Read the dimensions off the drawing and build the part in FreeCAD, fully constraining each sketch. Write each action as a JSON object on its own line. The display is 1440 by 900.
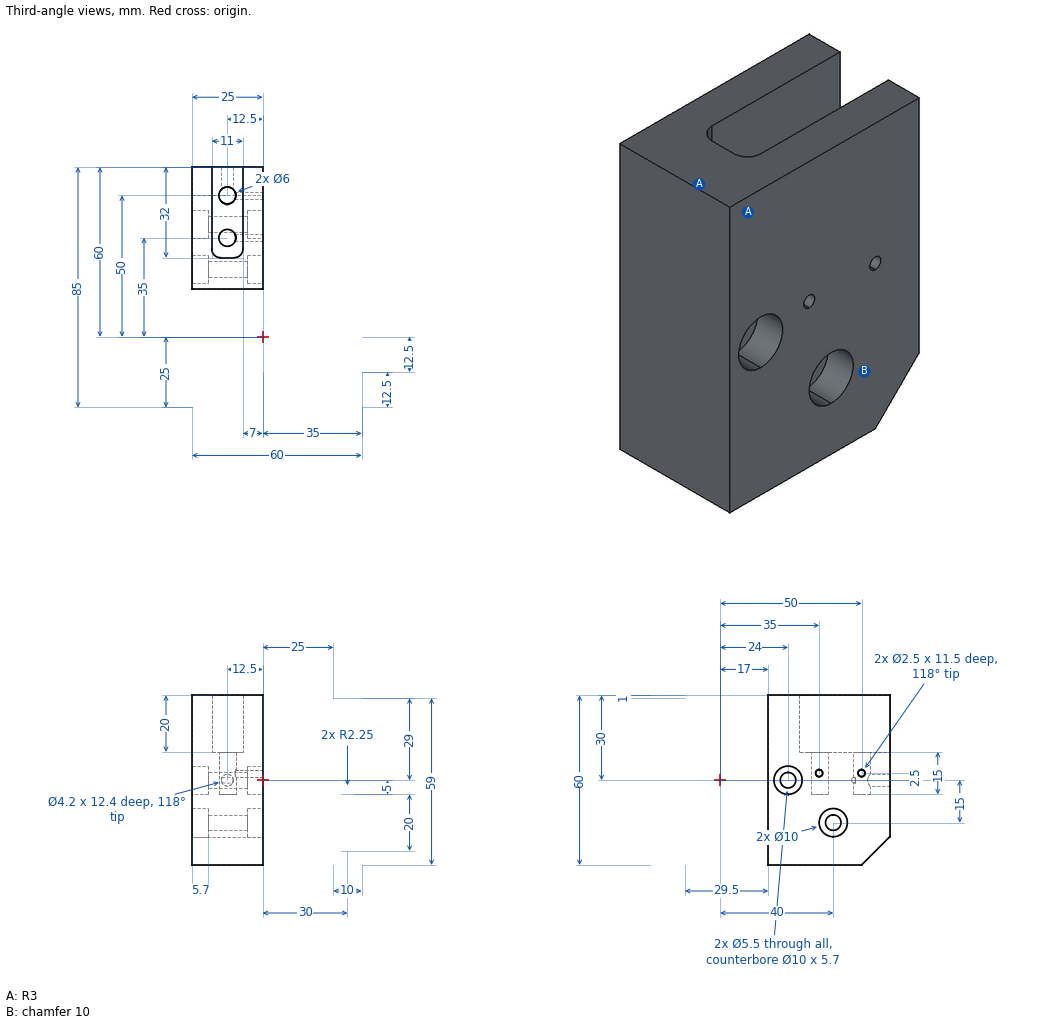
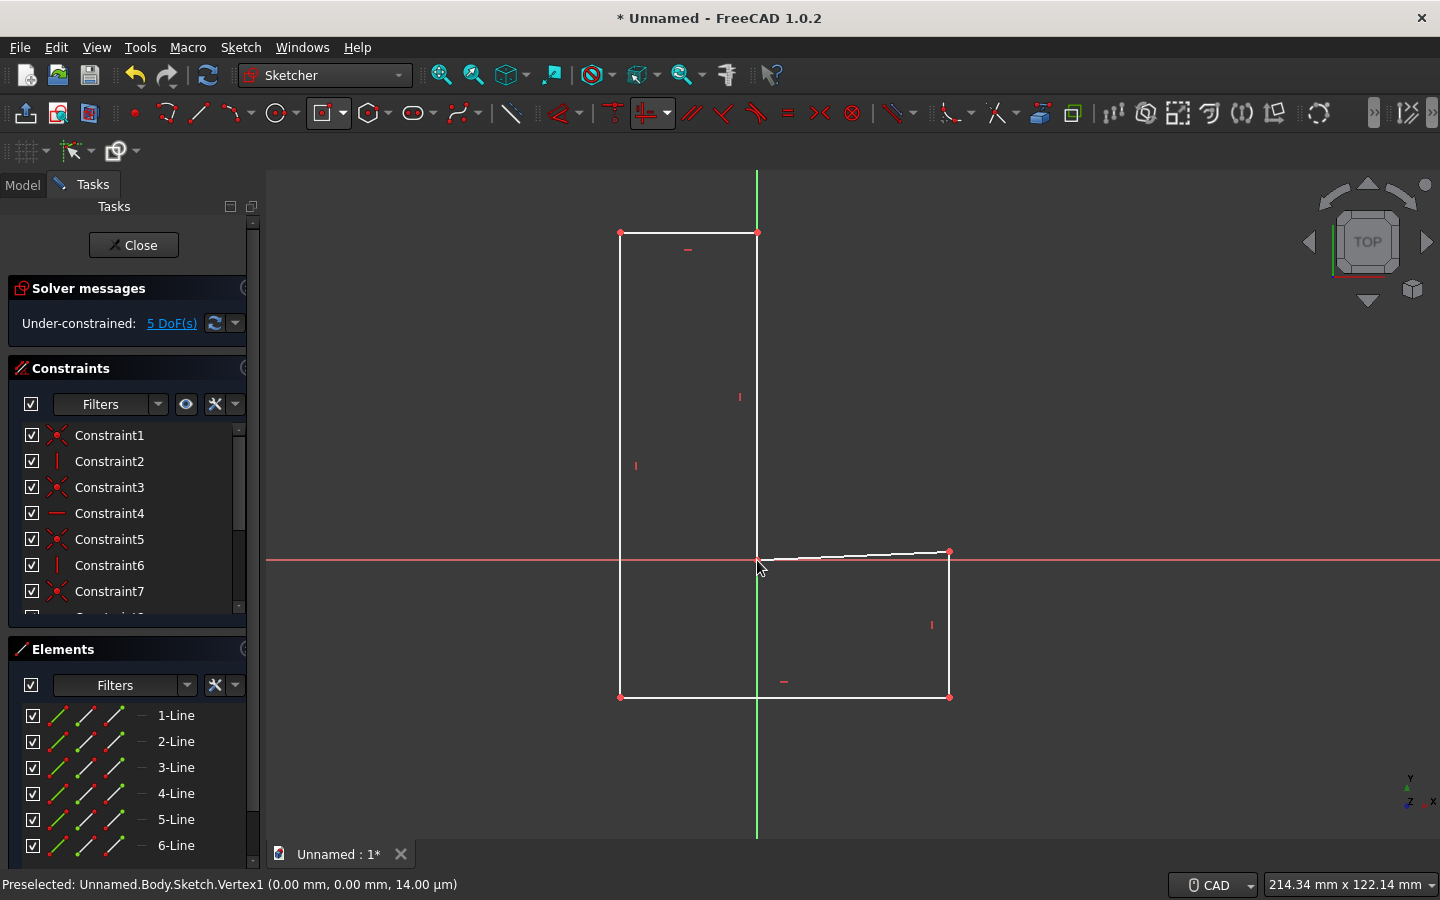
{"action": "left_click", "coordinate": [815, 558]}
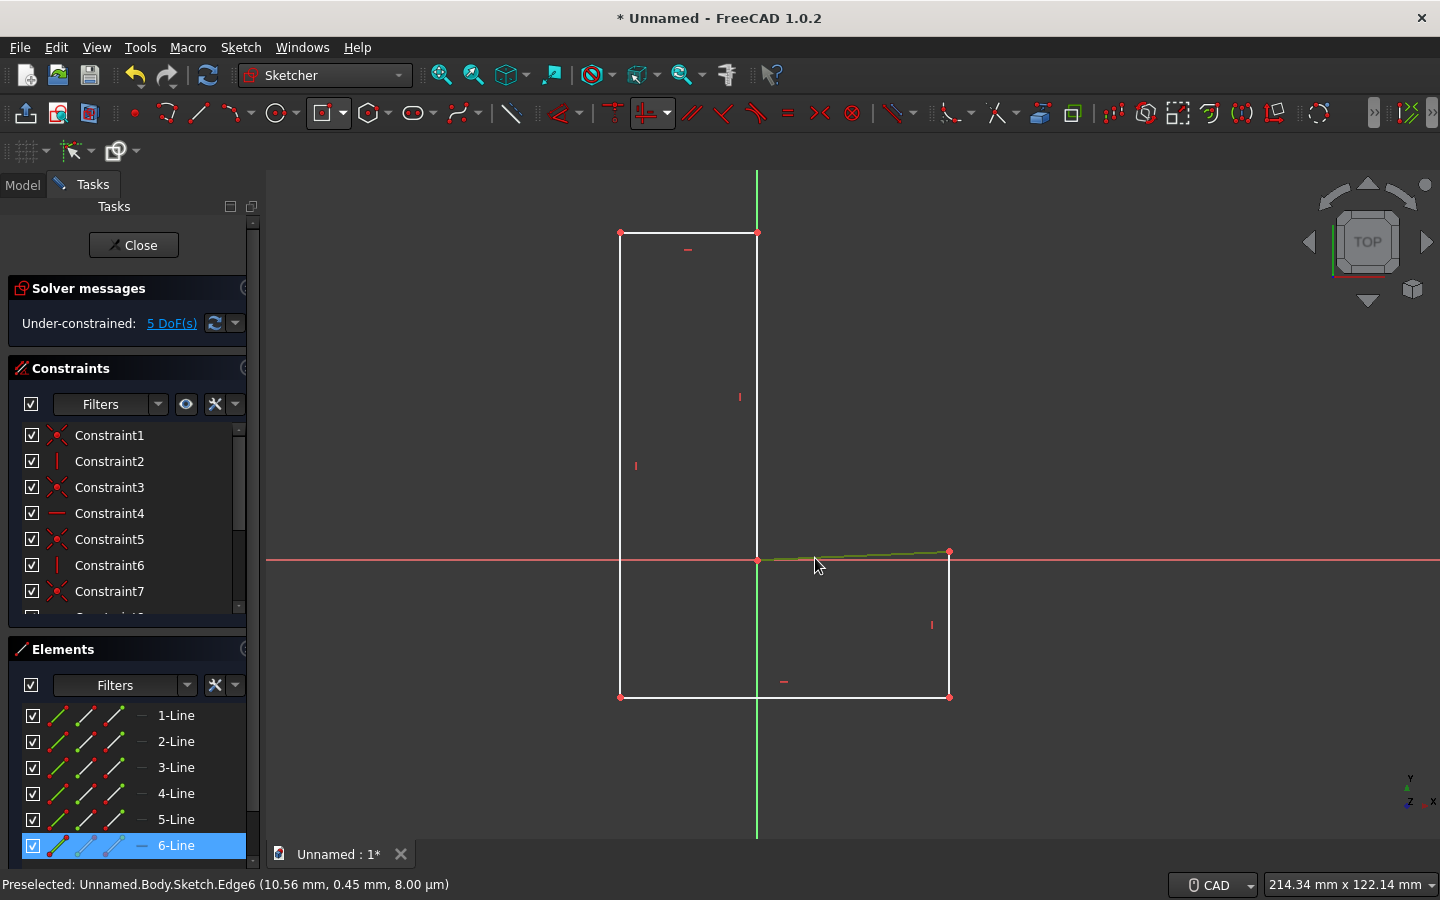
{"action": "key", "text": "h"}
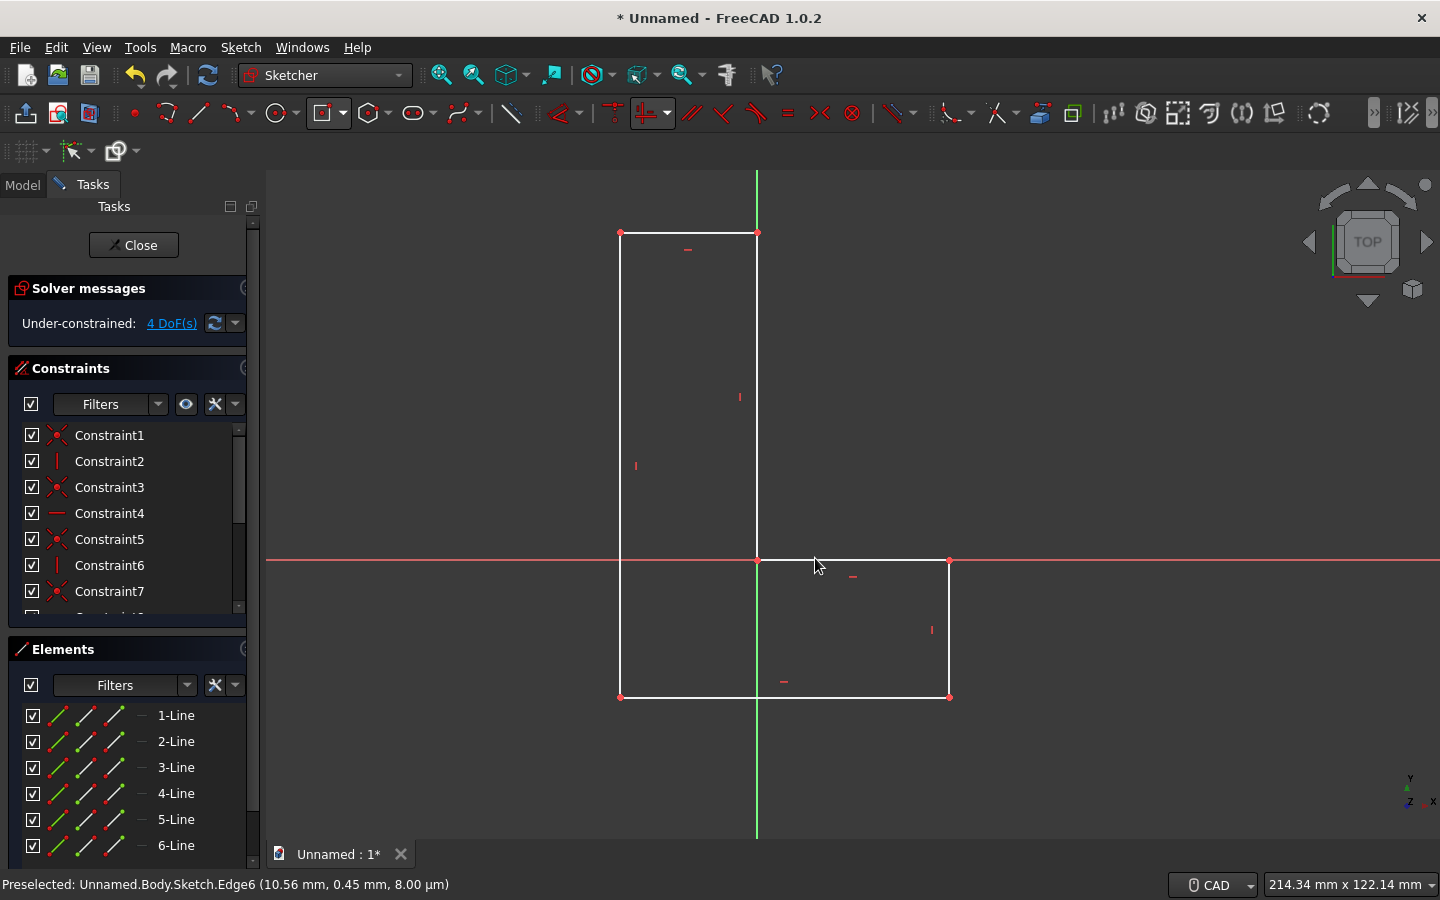
{"action": "left_click", "coordinate": [757, 462]}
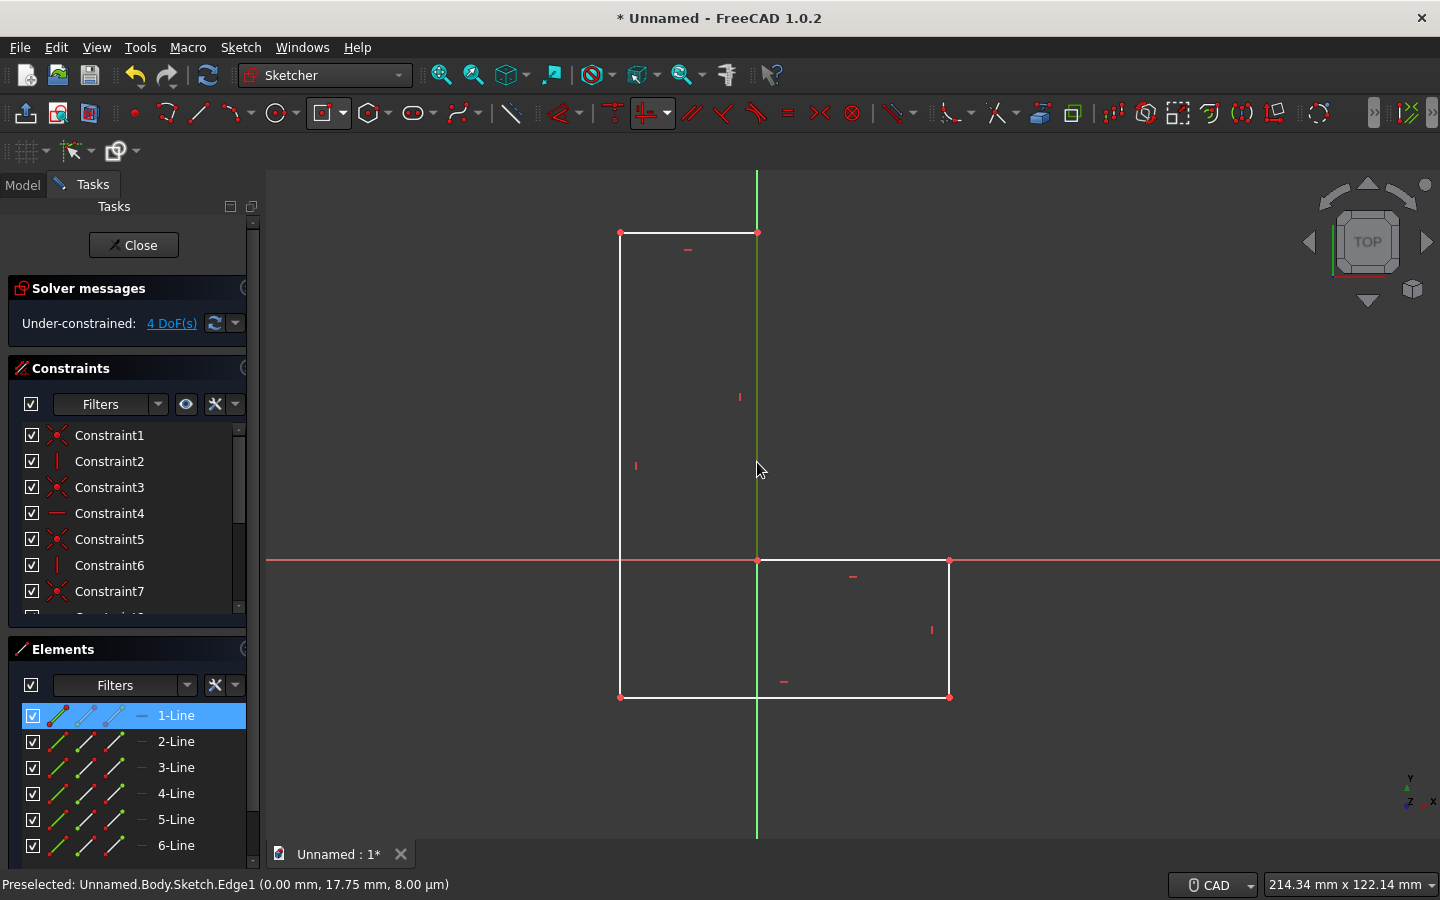
{"action": "left_click", "coordinate": [582, 114]}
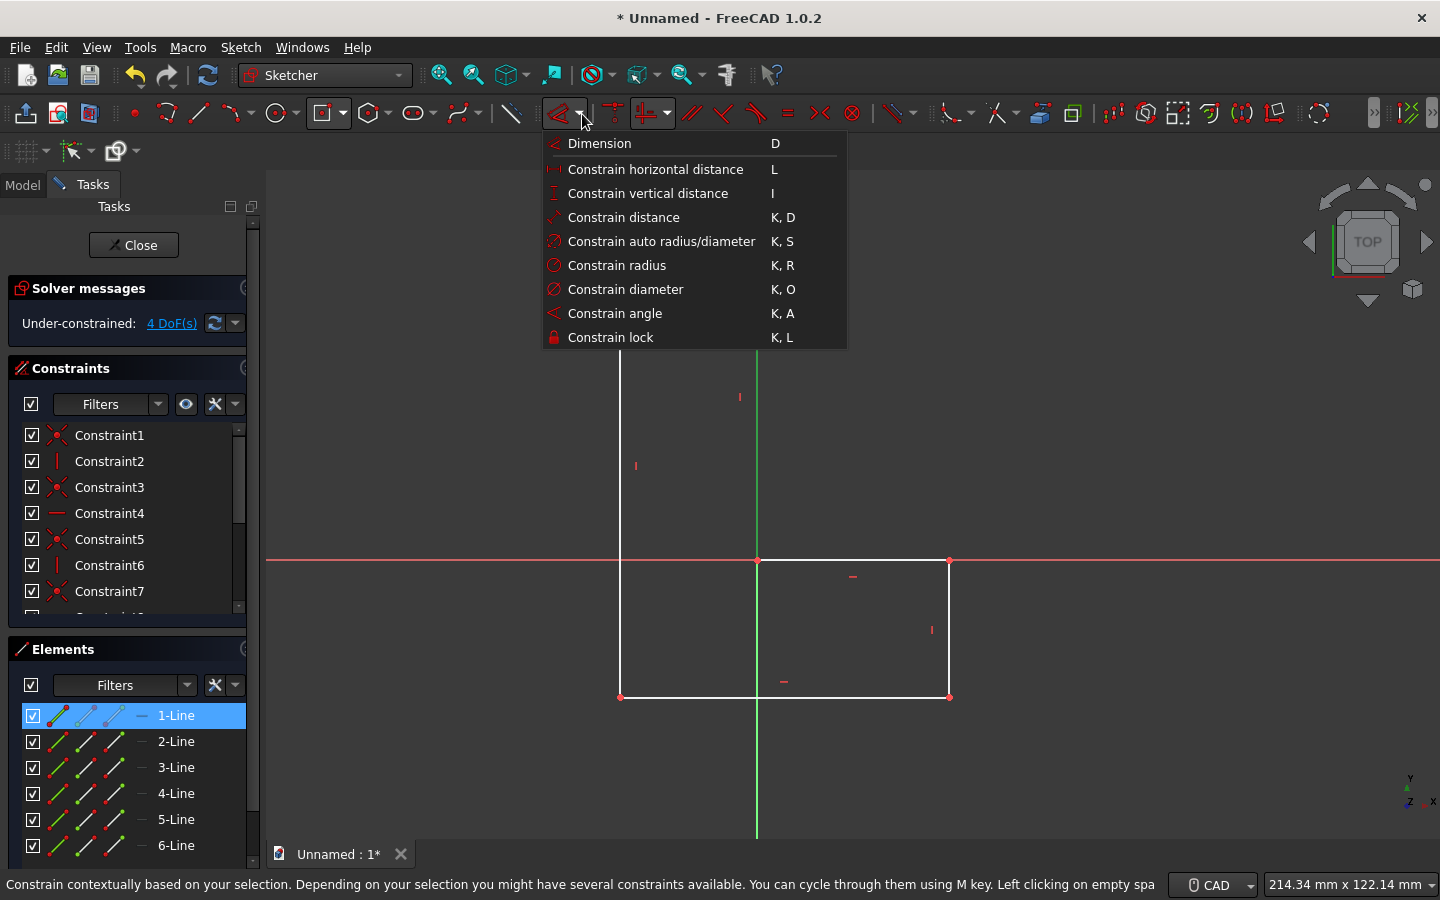
{"action": "left_click", "coordinate": [695, 193]}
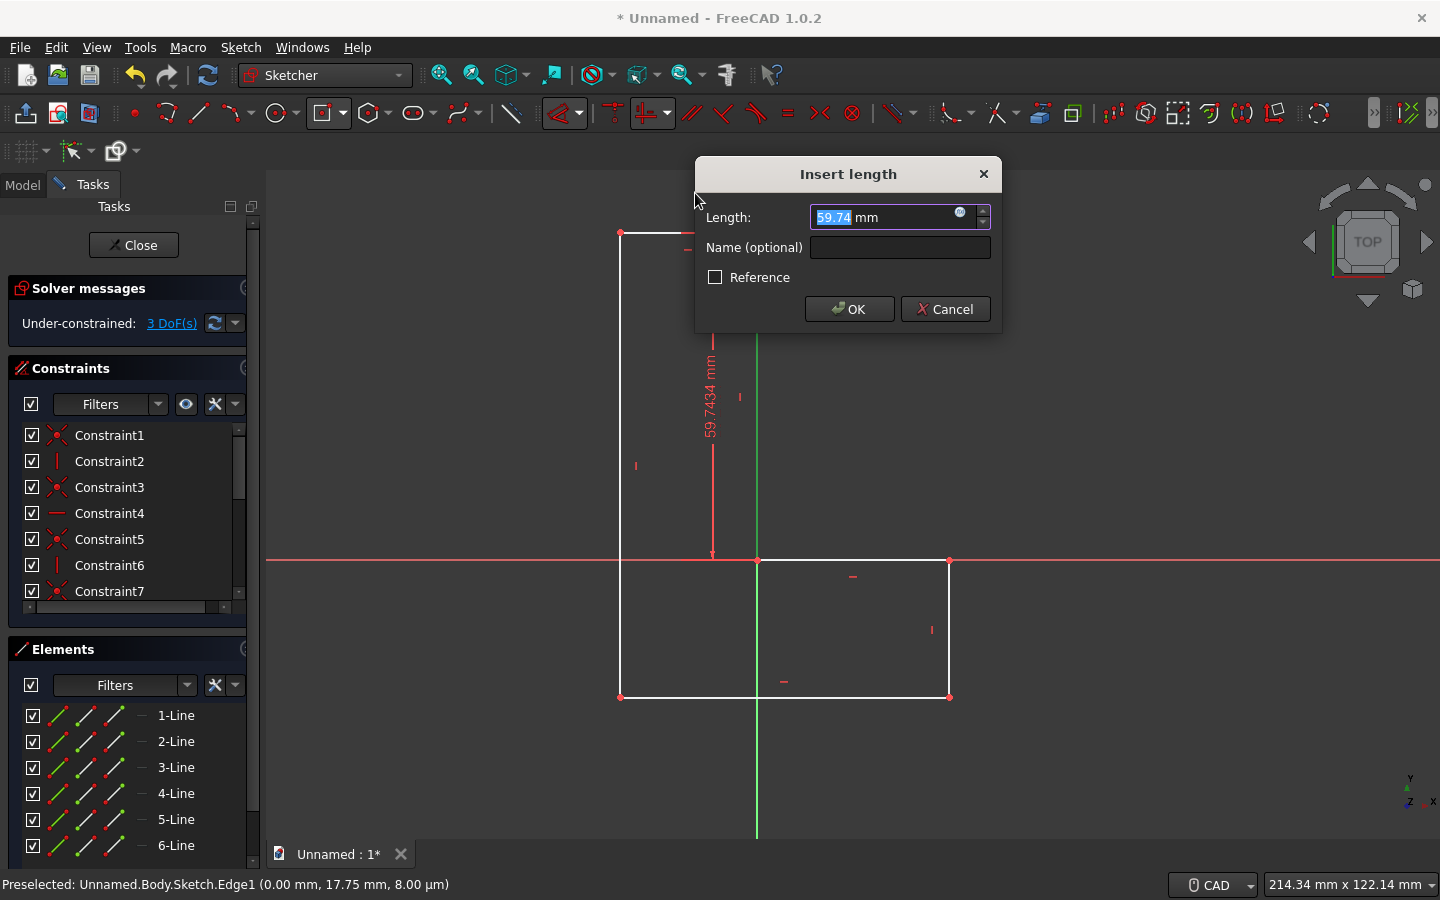
{"action": "type", "text": "60"}
{"action": "key", "text": "Return"}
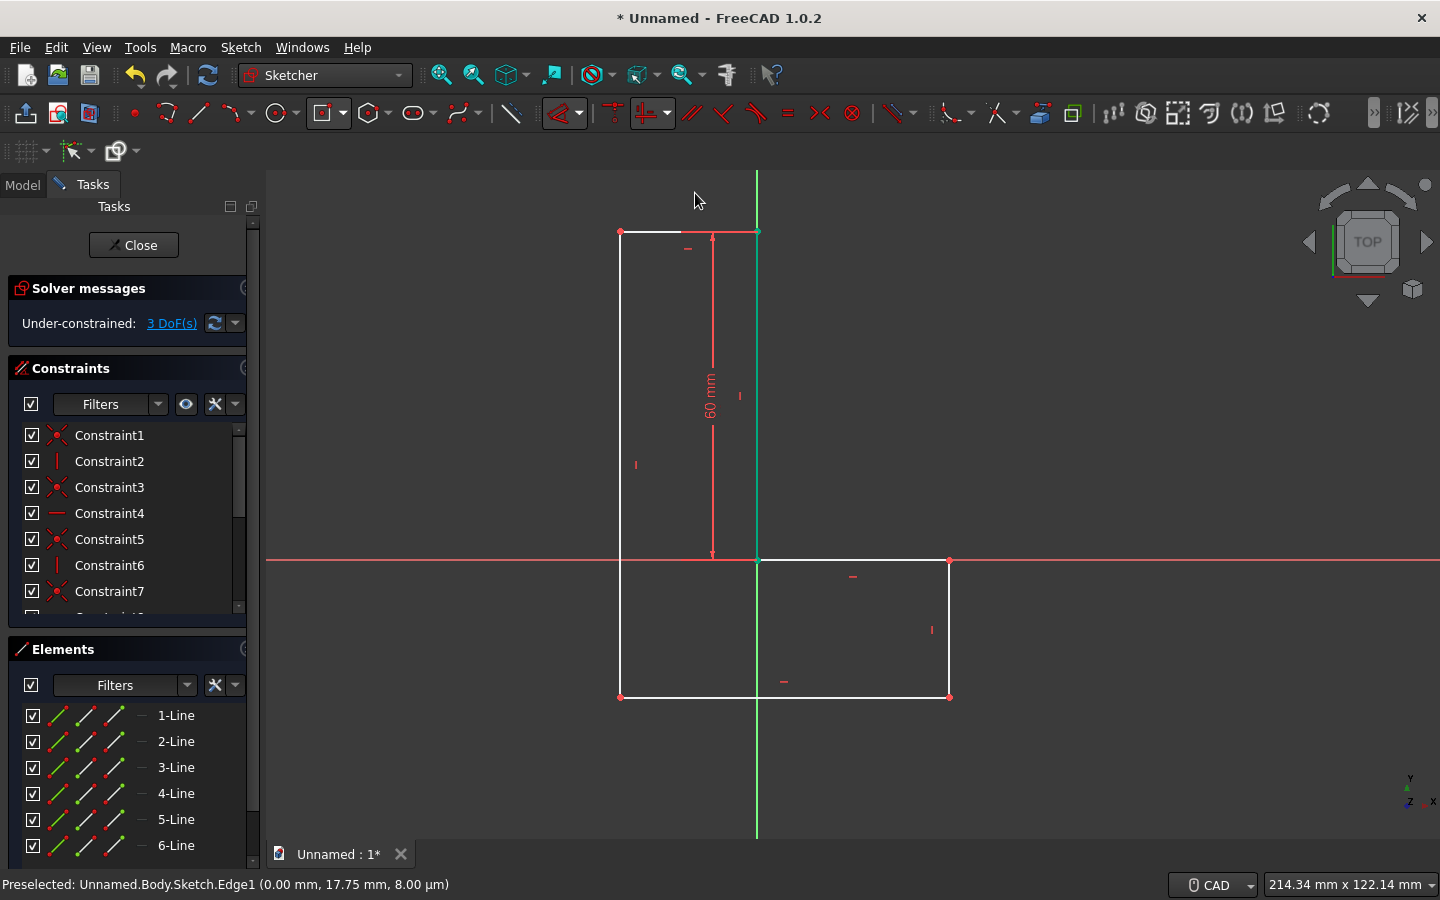
{"action": "left_click", "coordinate": [716, 232]}